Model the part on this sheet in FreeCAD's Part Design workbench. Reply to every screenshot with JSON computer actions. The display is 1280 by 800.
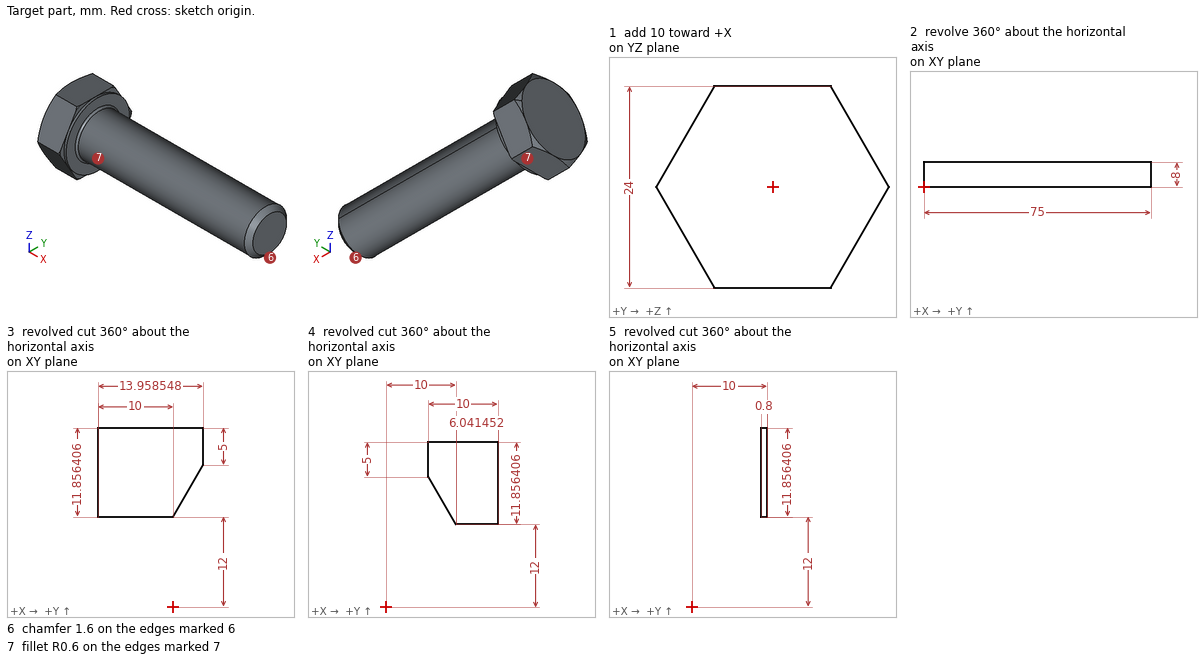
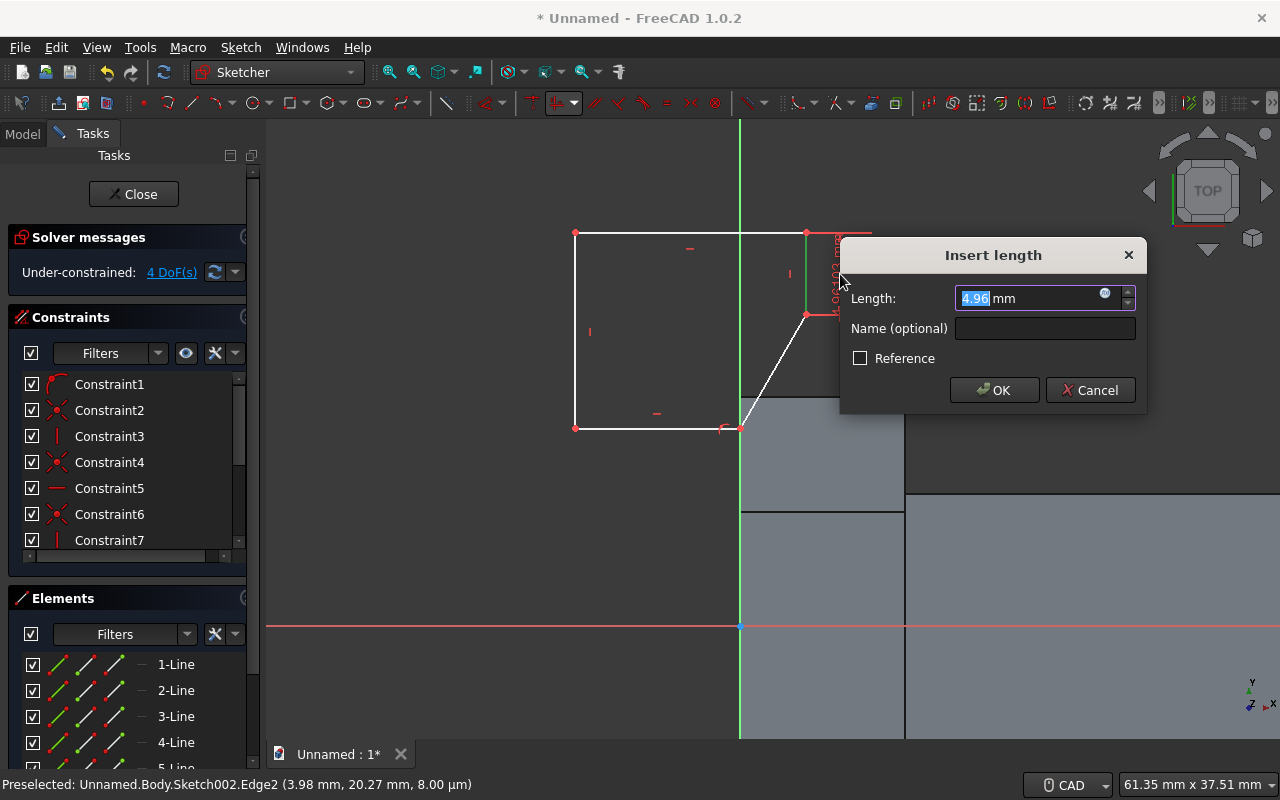
{"action": "type", "text": "5"}
{"action": "key", "text": "Return"}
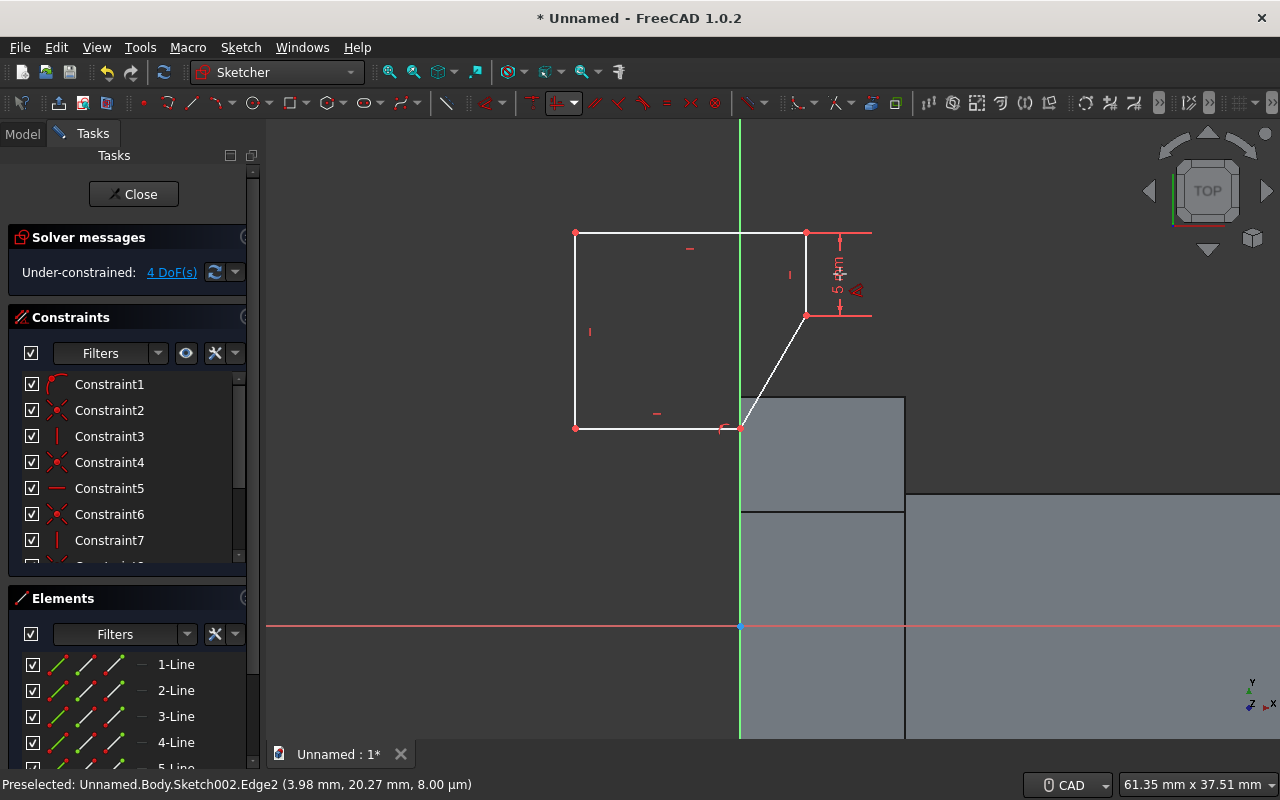
{"action": "left_click", "coordinate": [625, 429]}
{"action": "left_click", "coordinate": [658, 463]}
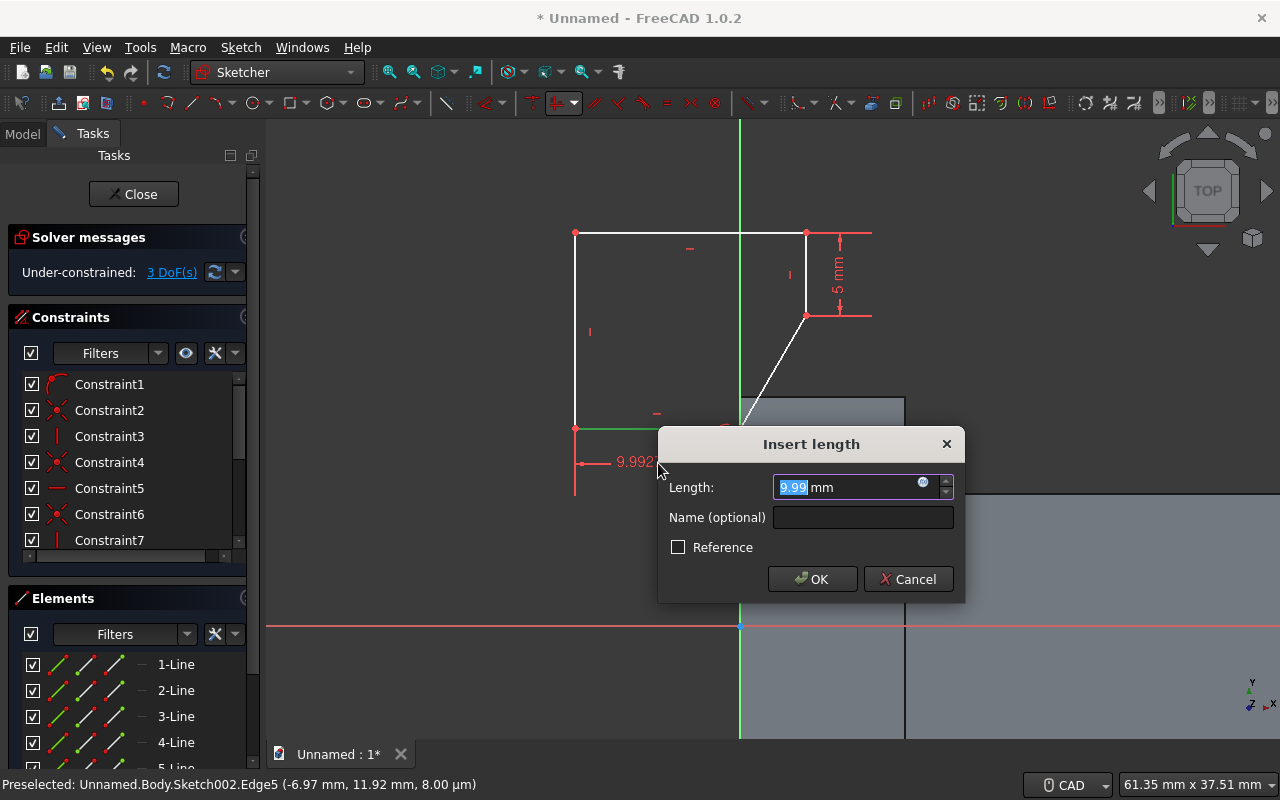
{"action": "type", "text": "10"}
{"action": "key", "text": "Return"}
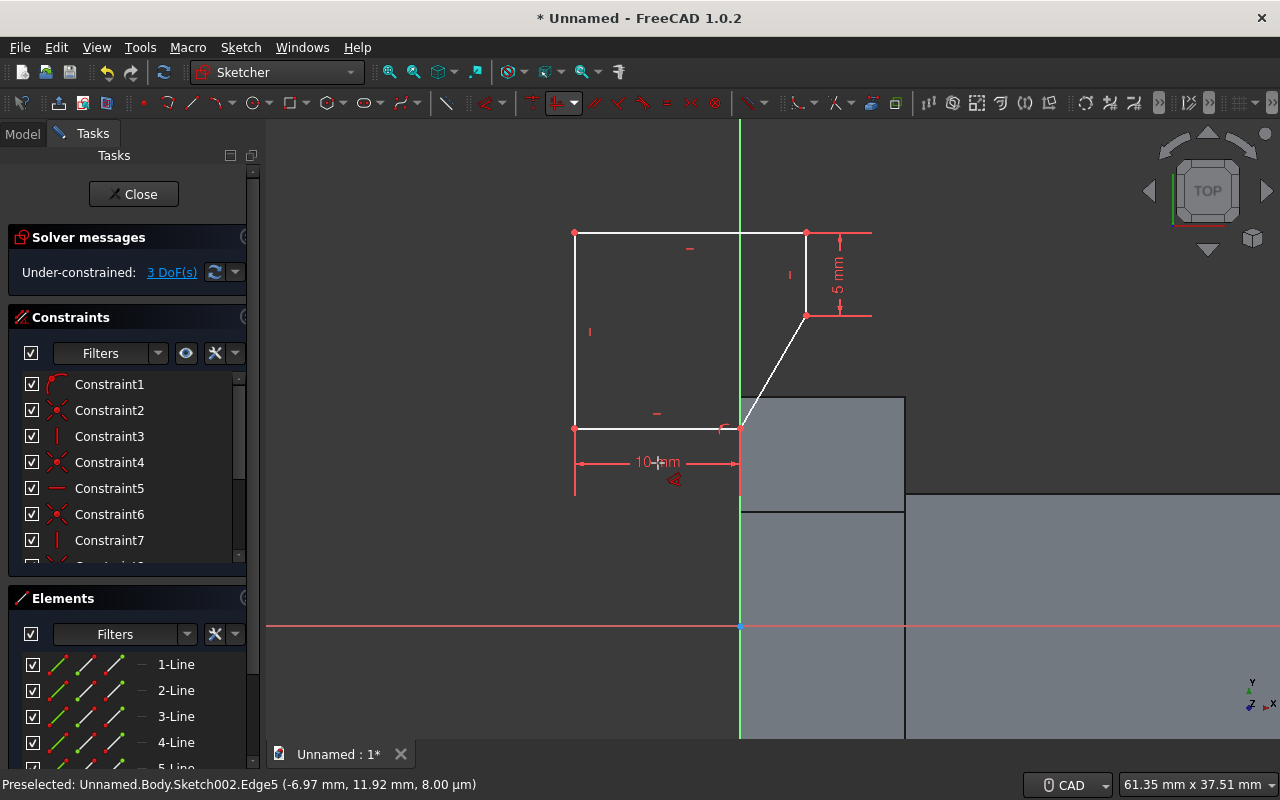
{"action": "left_click", "coordinate": [740, 429]}
{"action": "left_click", "coordinate": [774, 528]}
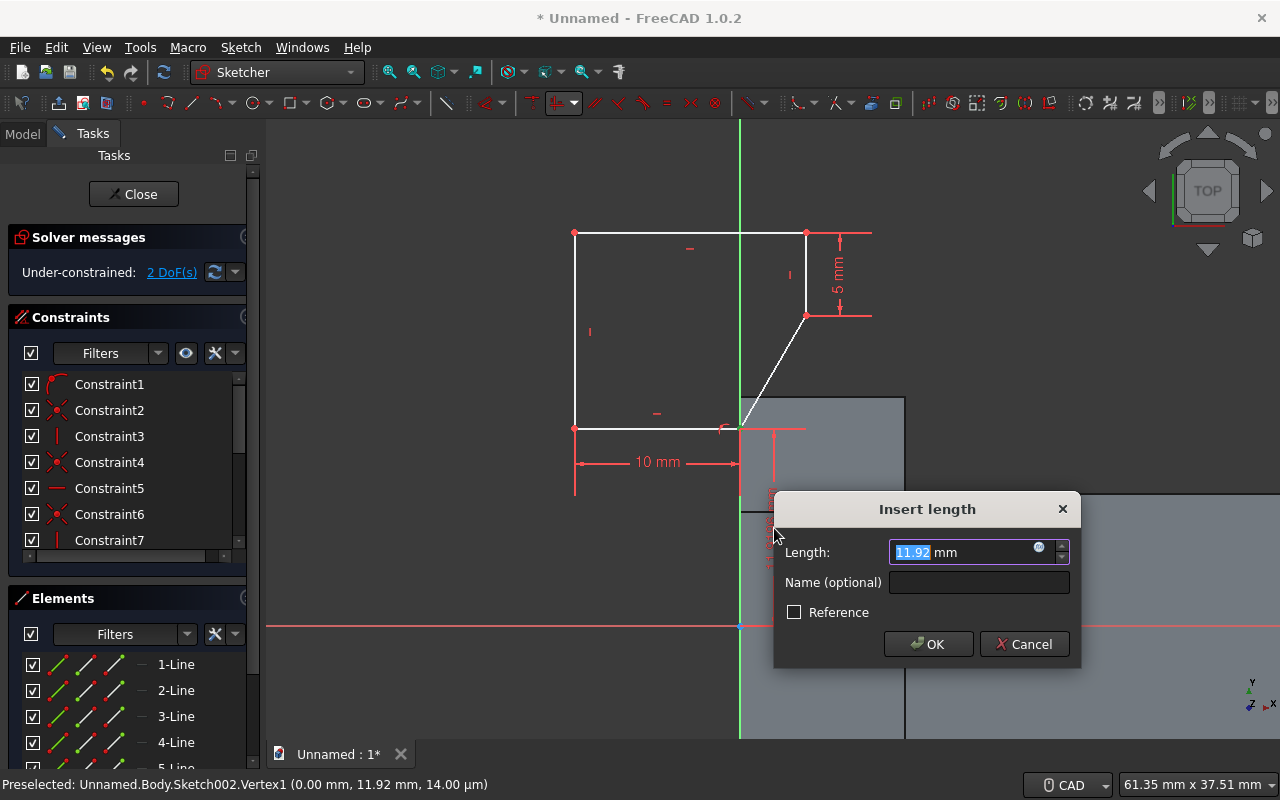
{"action": "type", "text": "12"}
{"action": "key", "text": "Return"}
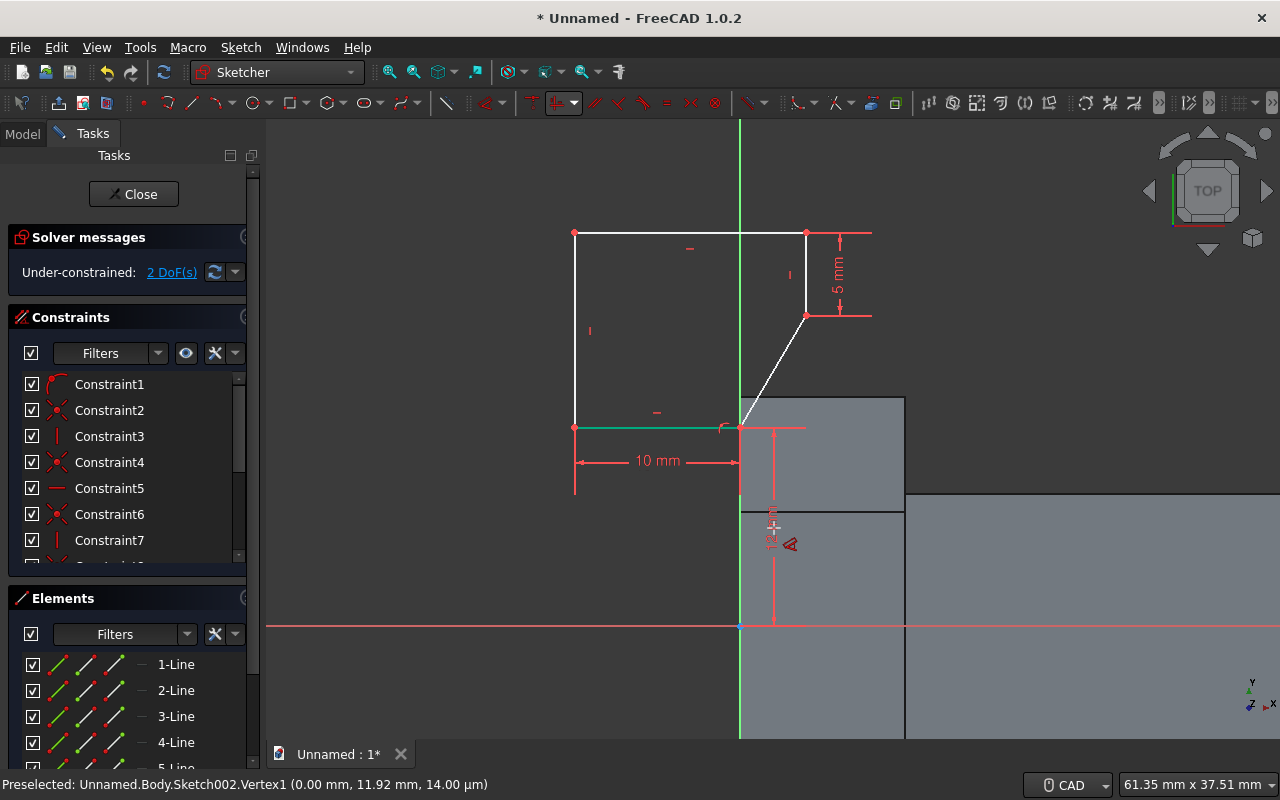
{"action": "left_click", "coordinate": [737, 233]}
{"action": "left_click", "coordinate": [690, 199]}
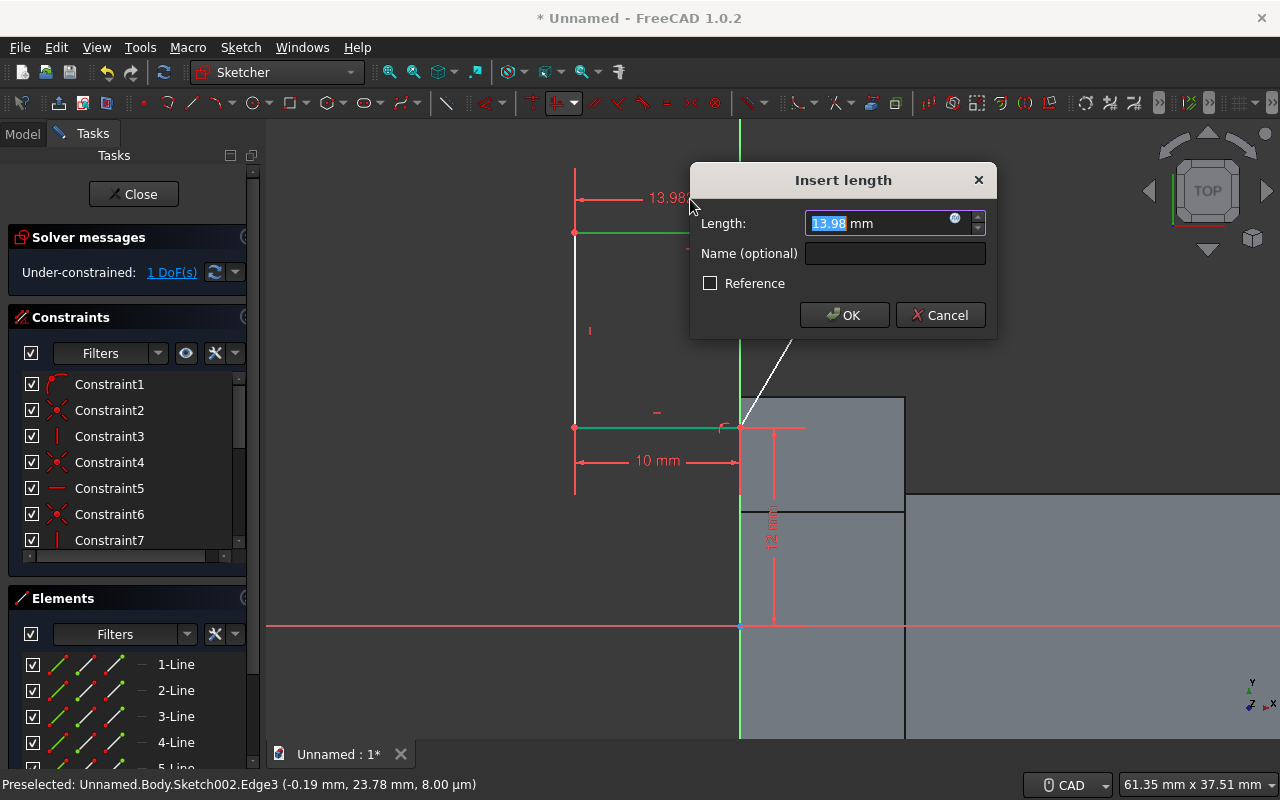
{"action": "type", "text": "13.958548"}
{"action": "key", "text": "Return"}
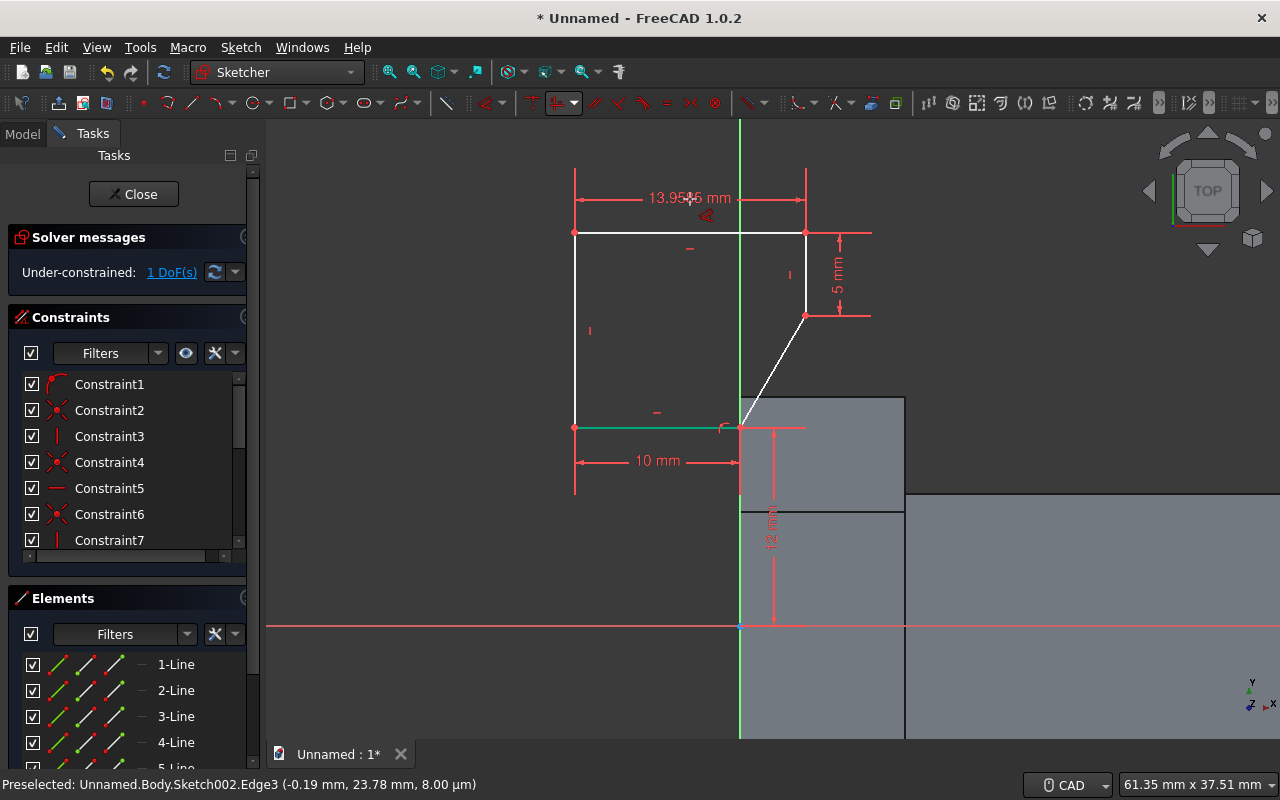
{"action": "left_click", "coordinate": [575, 291]}
{"action": "left_click", "coordinate": [541, 330]}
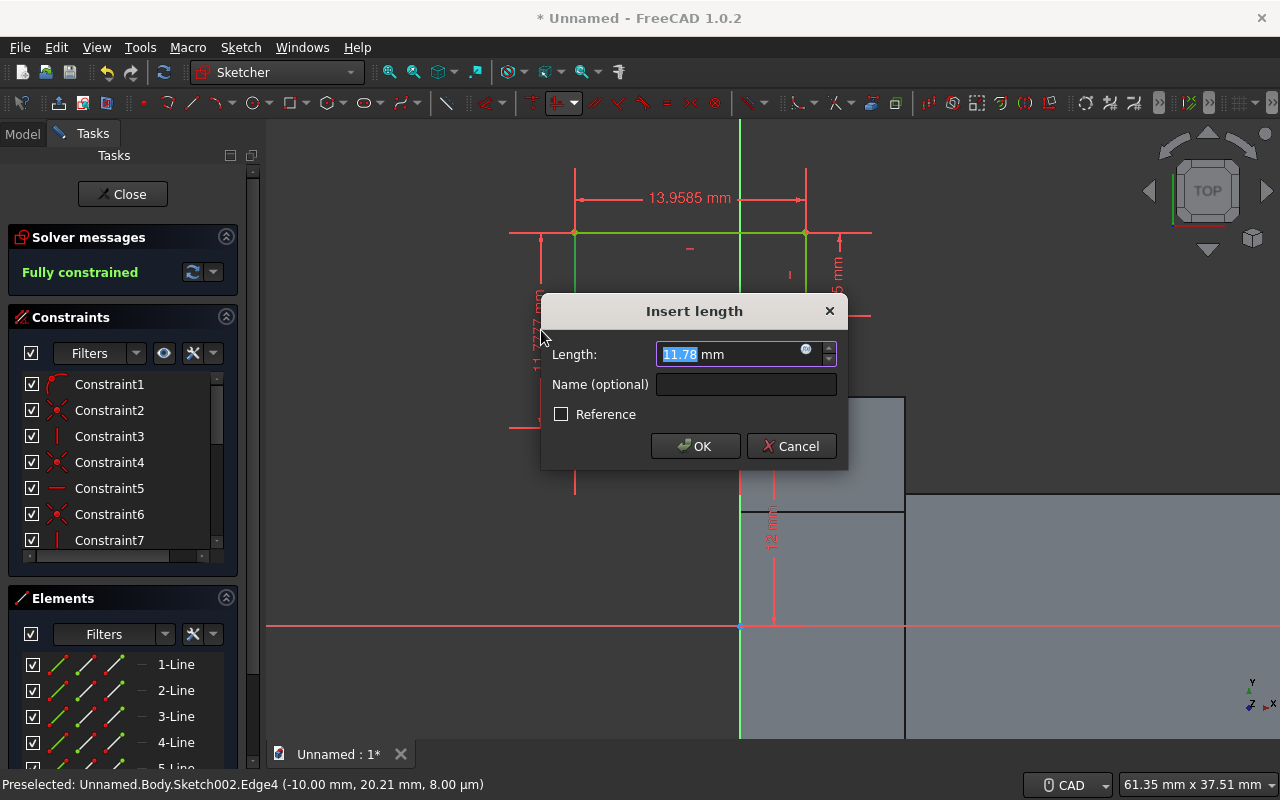
{"action": "type", "text": "11.856406"}
{"action": "key", "text": "Return"}
{"action": "key", "text": "Escape"}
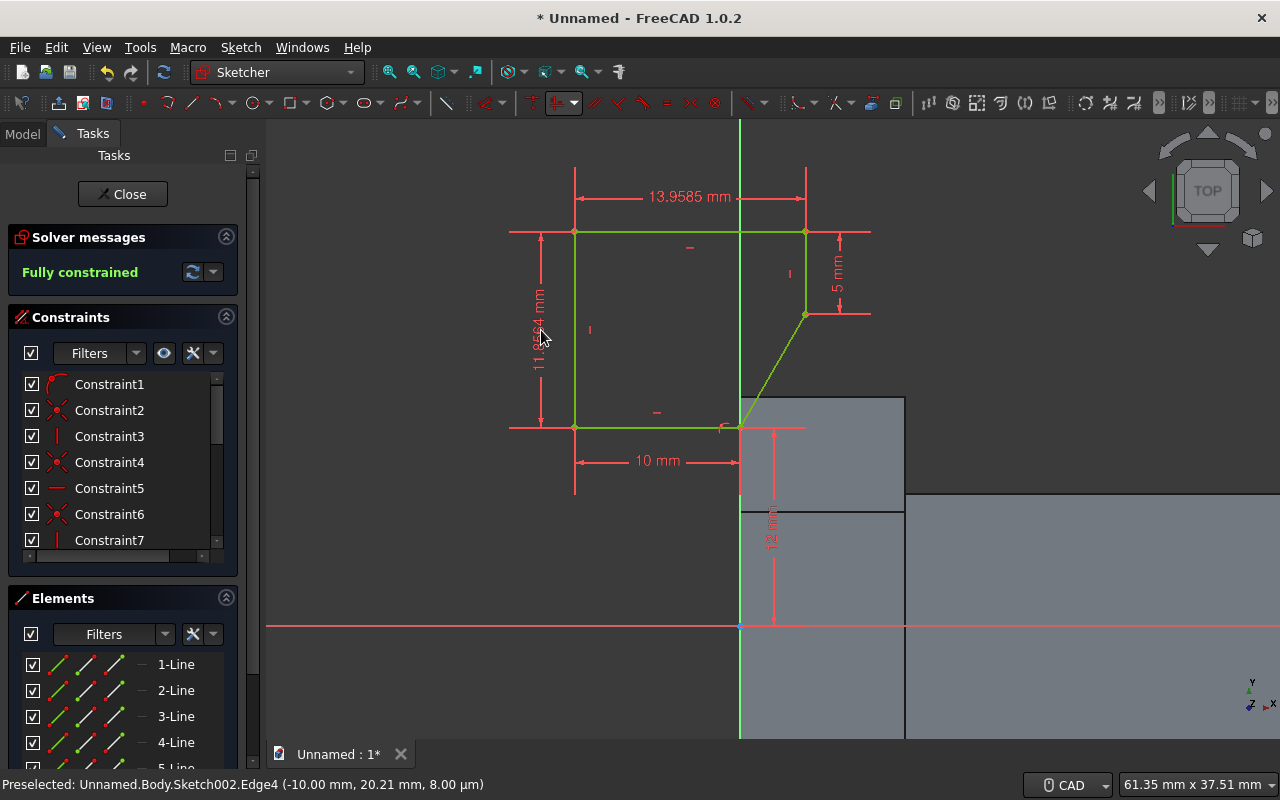
{"action": "left_click", "coordinate": [123, 194]}